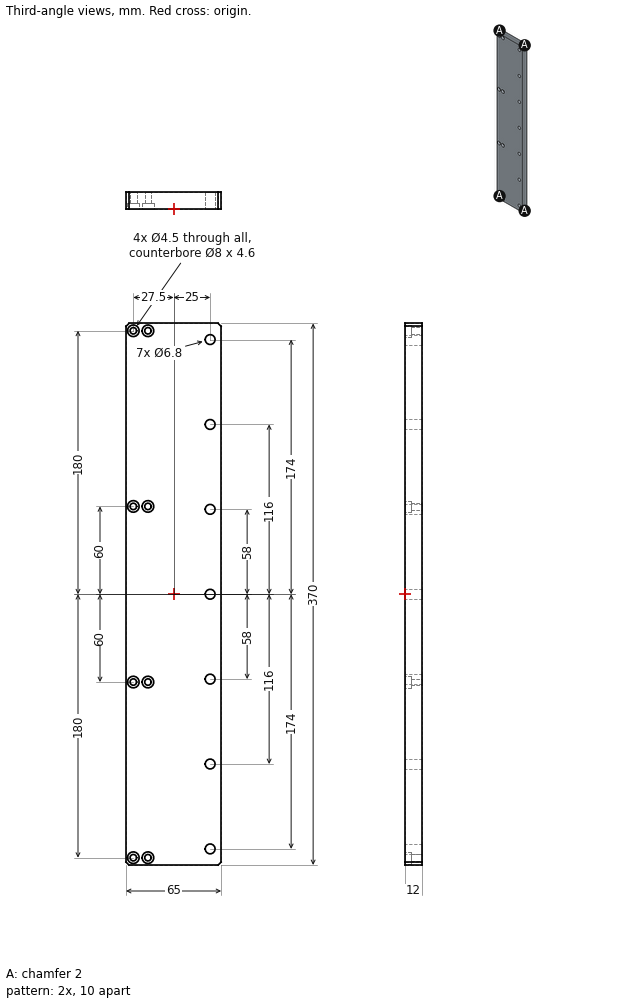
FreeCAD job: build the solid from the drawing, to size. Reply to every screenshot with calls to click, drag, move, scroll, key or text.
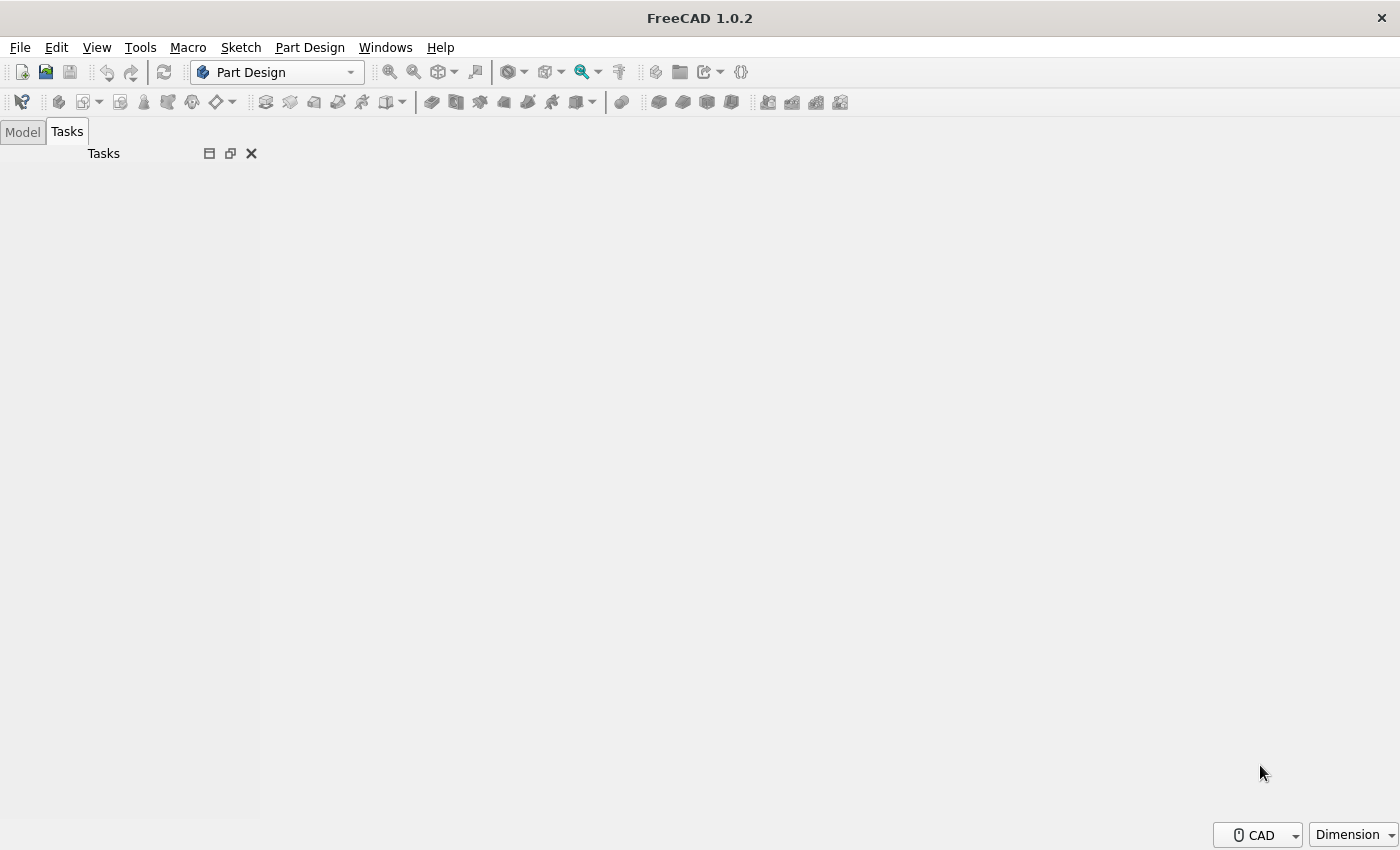
key(ctrl+n)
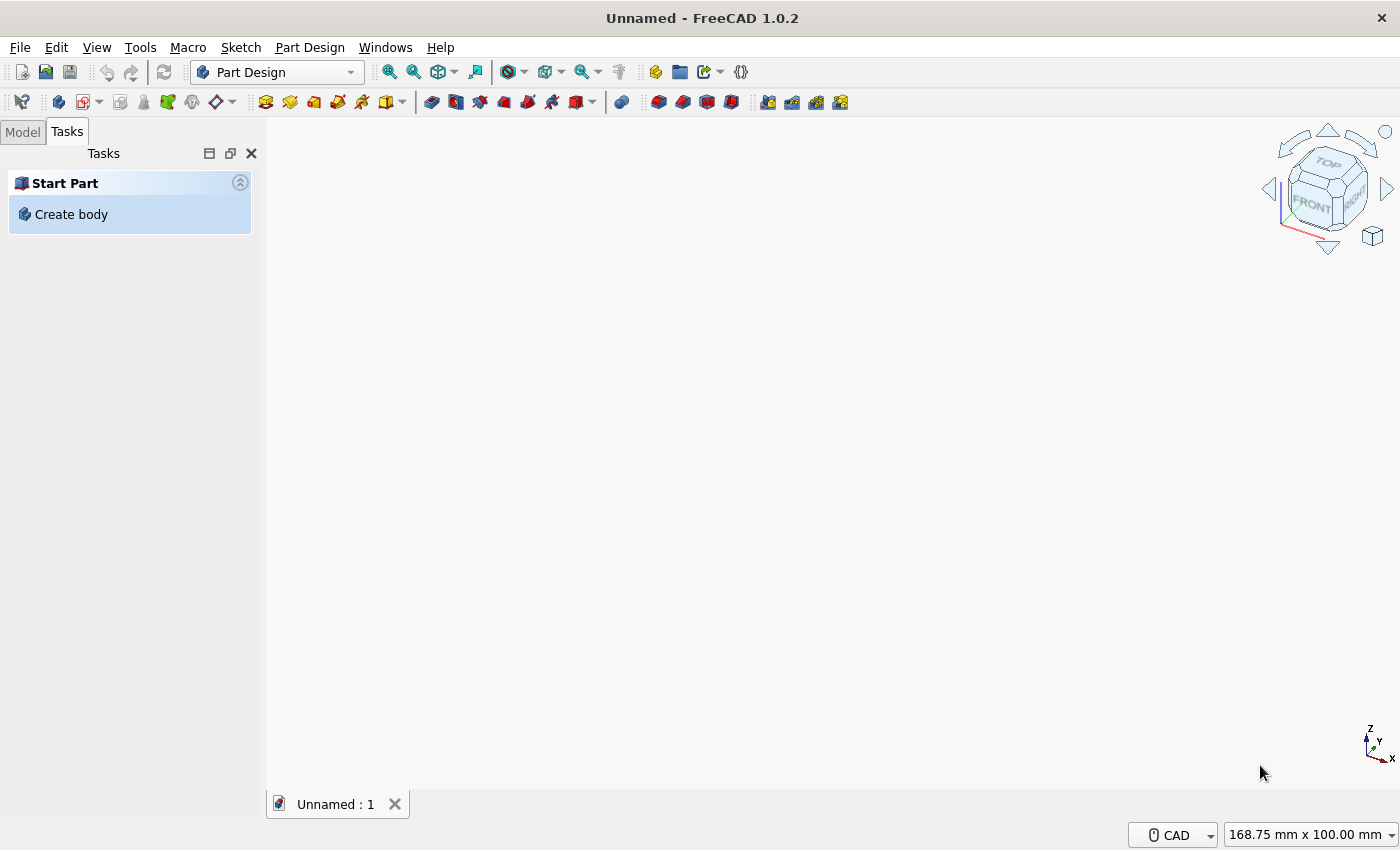
click(84, 102)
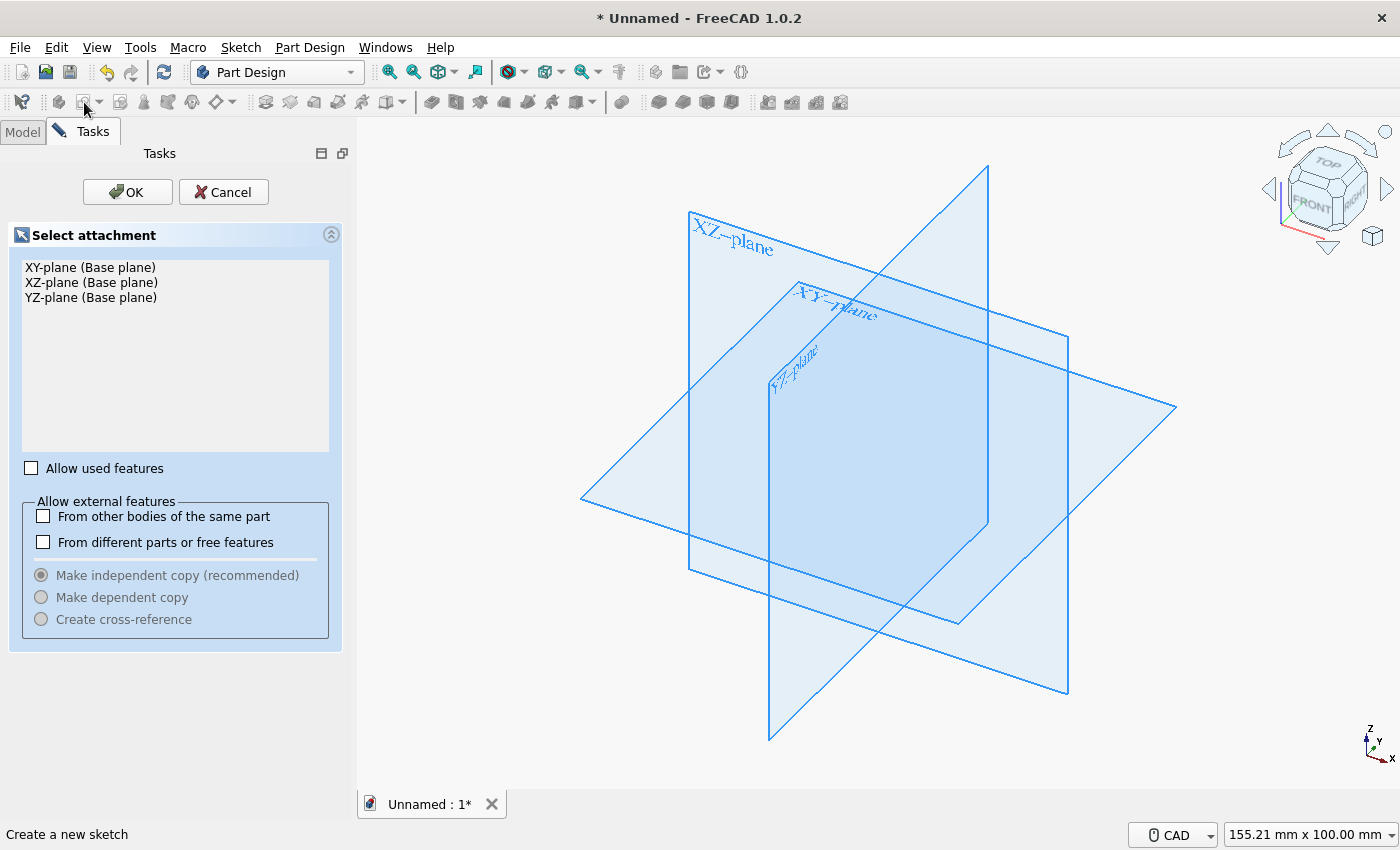
click(82, 282)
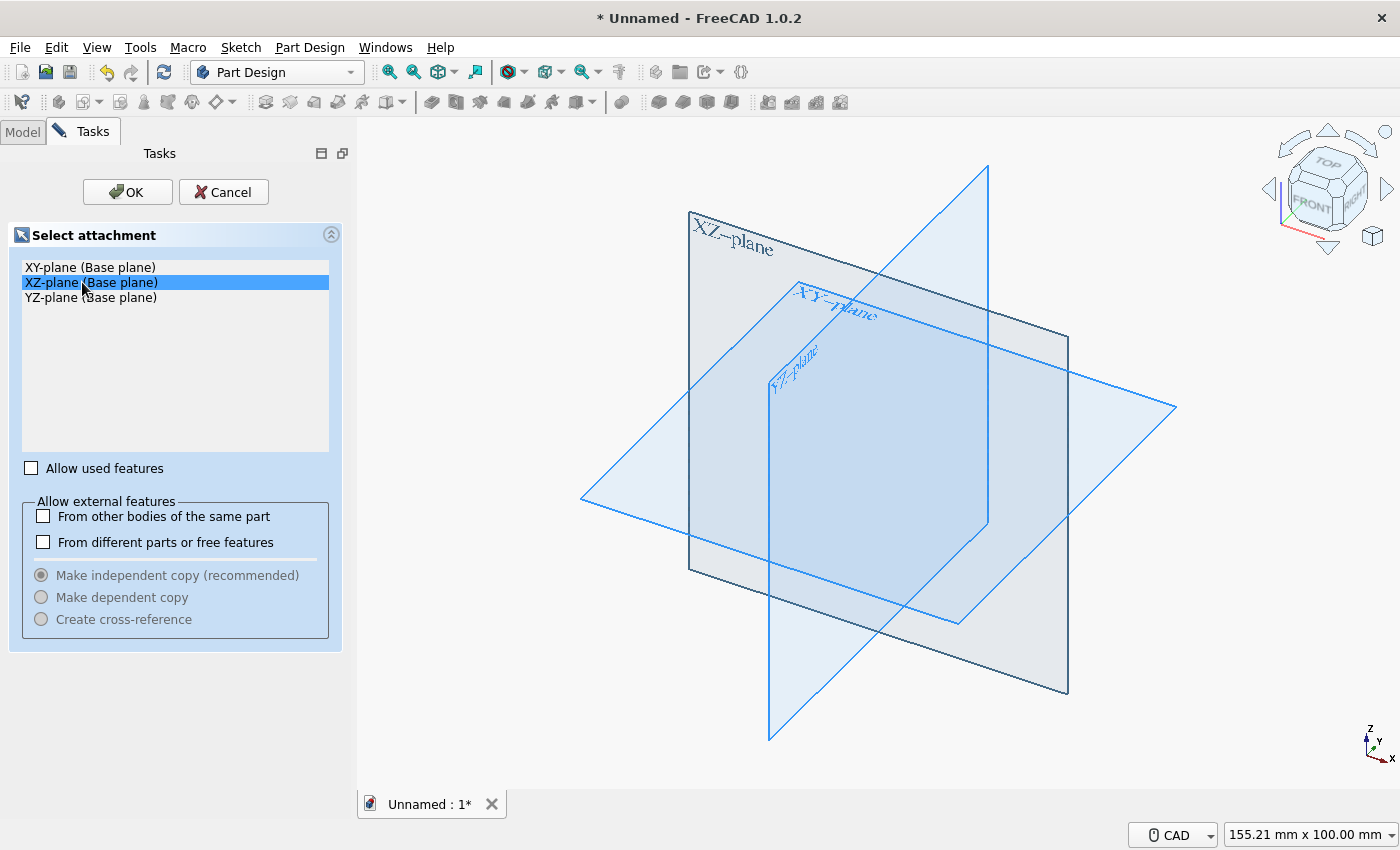
click(128, 192)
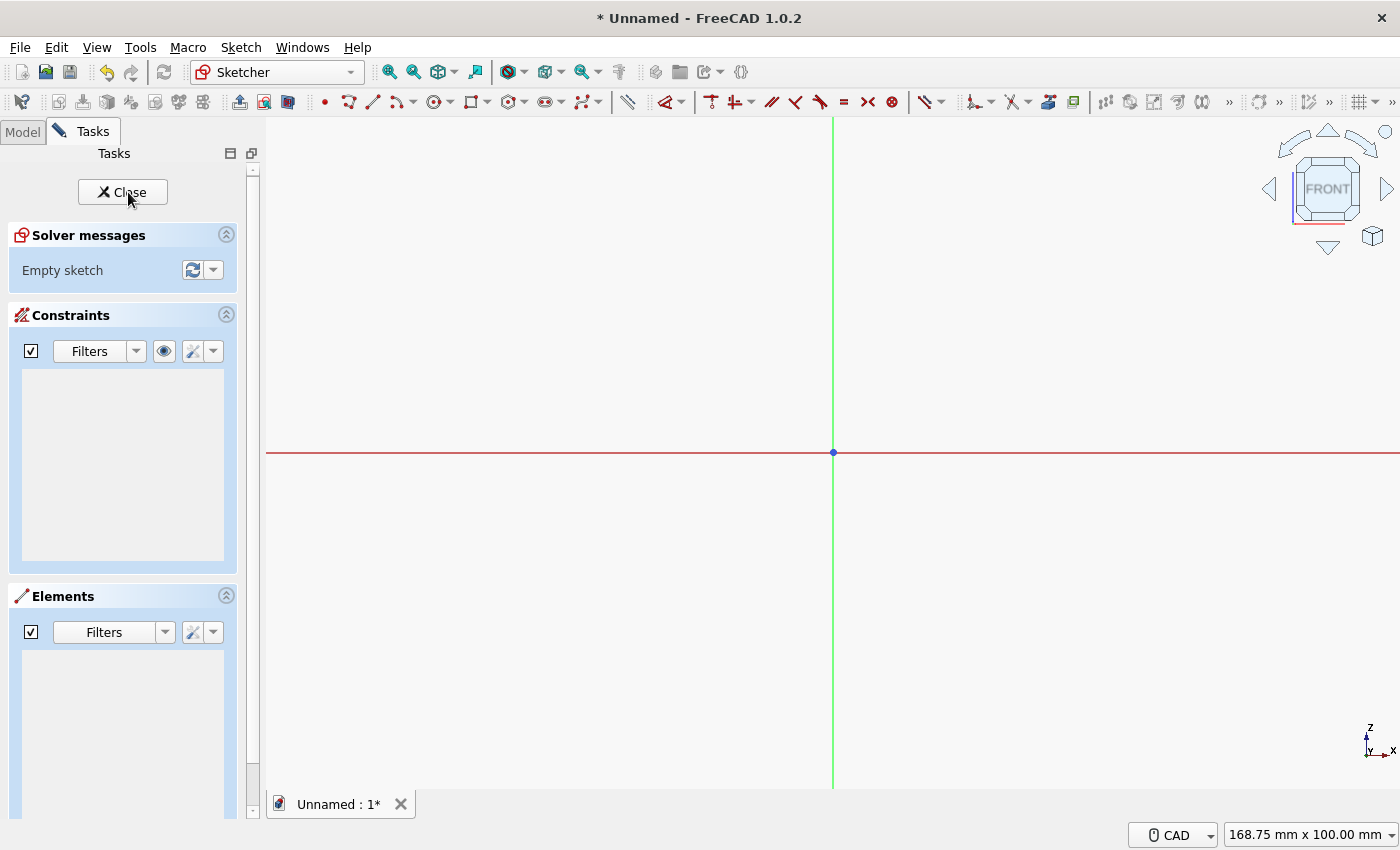
scroll(751, 453, down, 9)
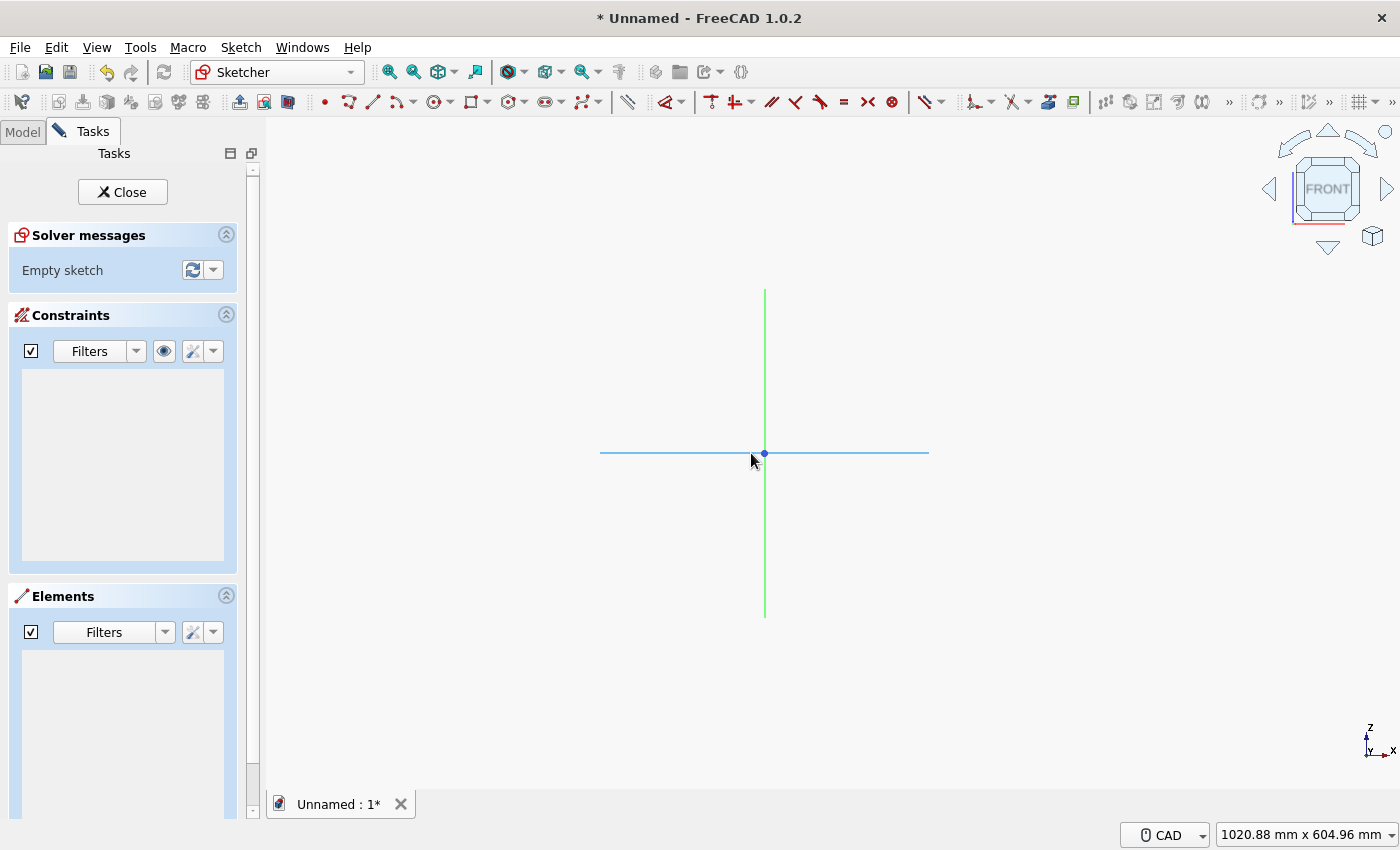
key(g)
key(v)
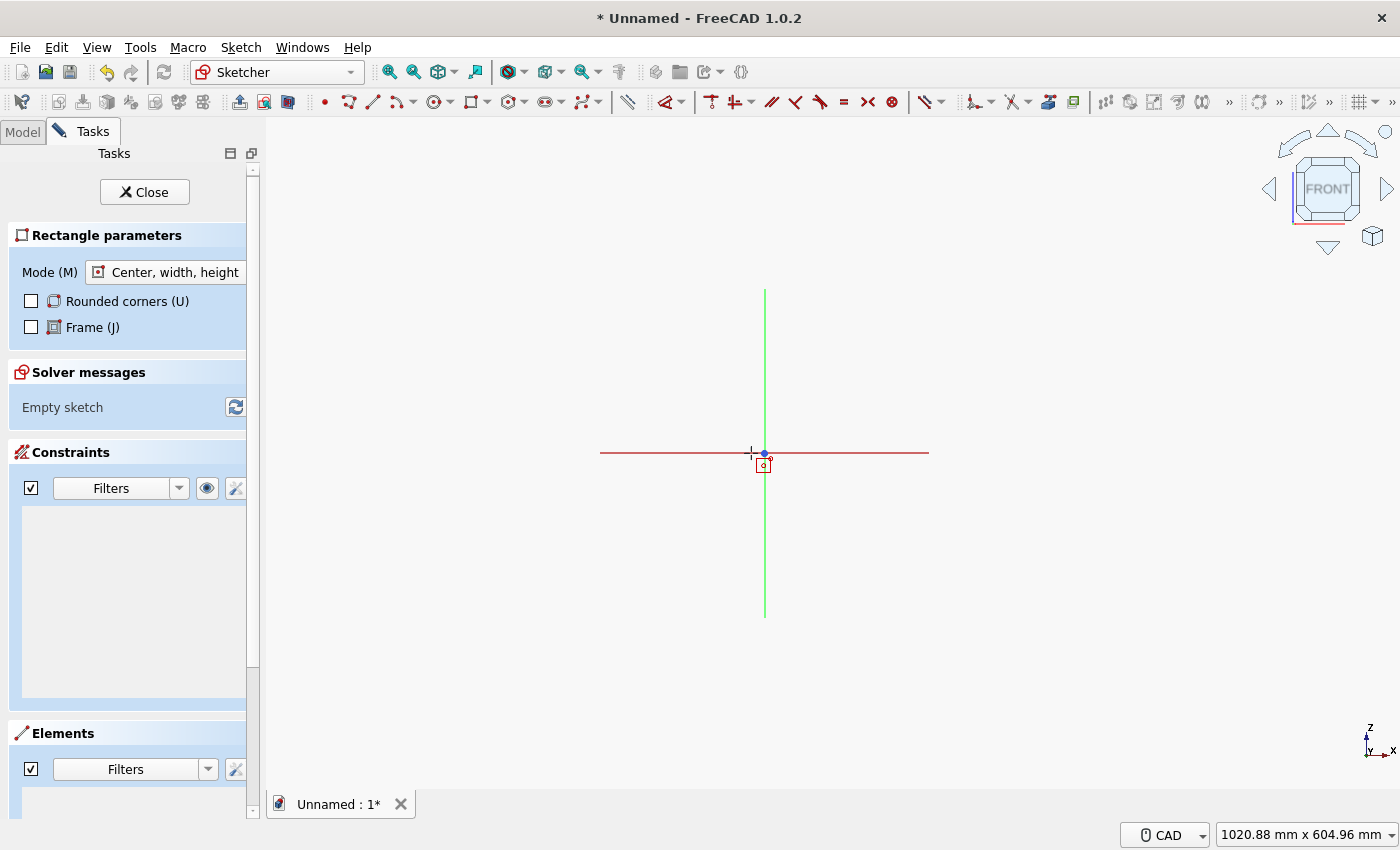
click(765, 453)
move(801, 248)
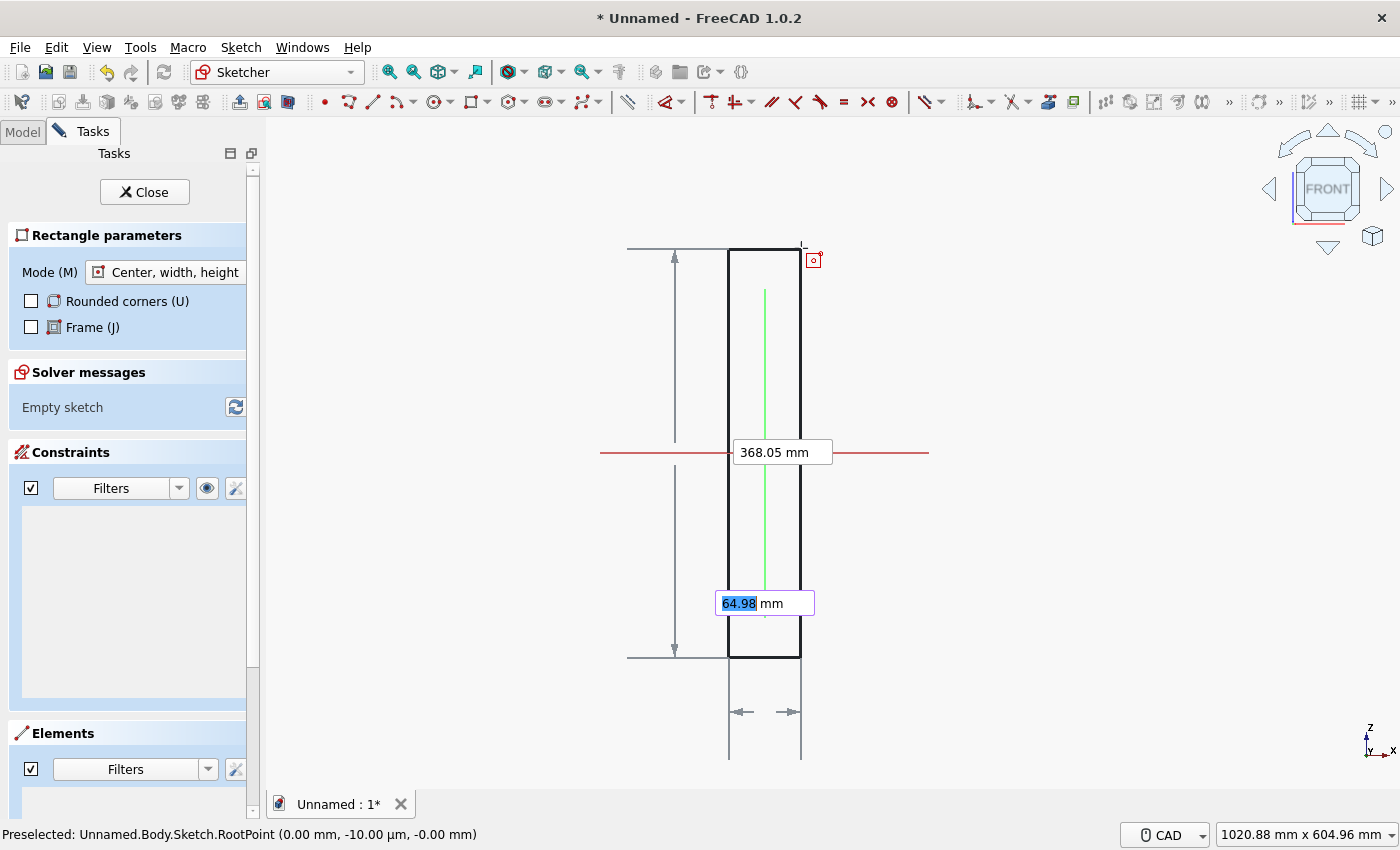
text(65)
key(Tab)
text(370)
key(Return)
key(Escape)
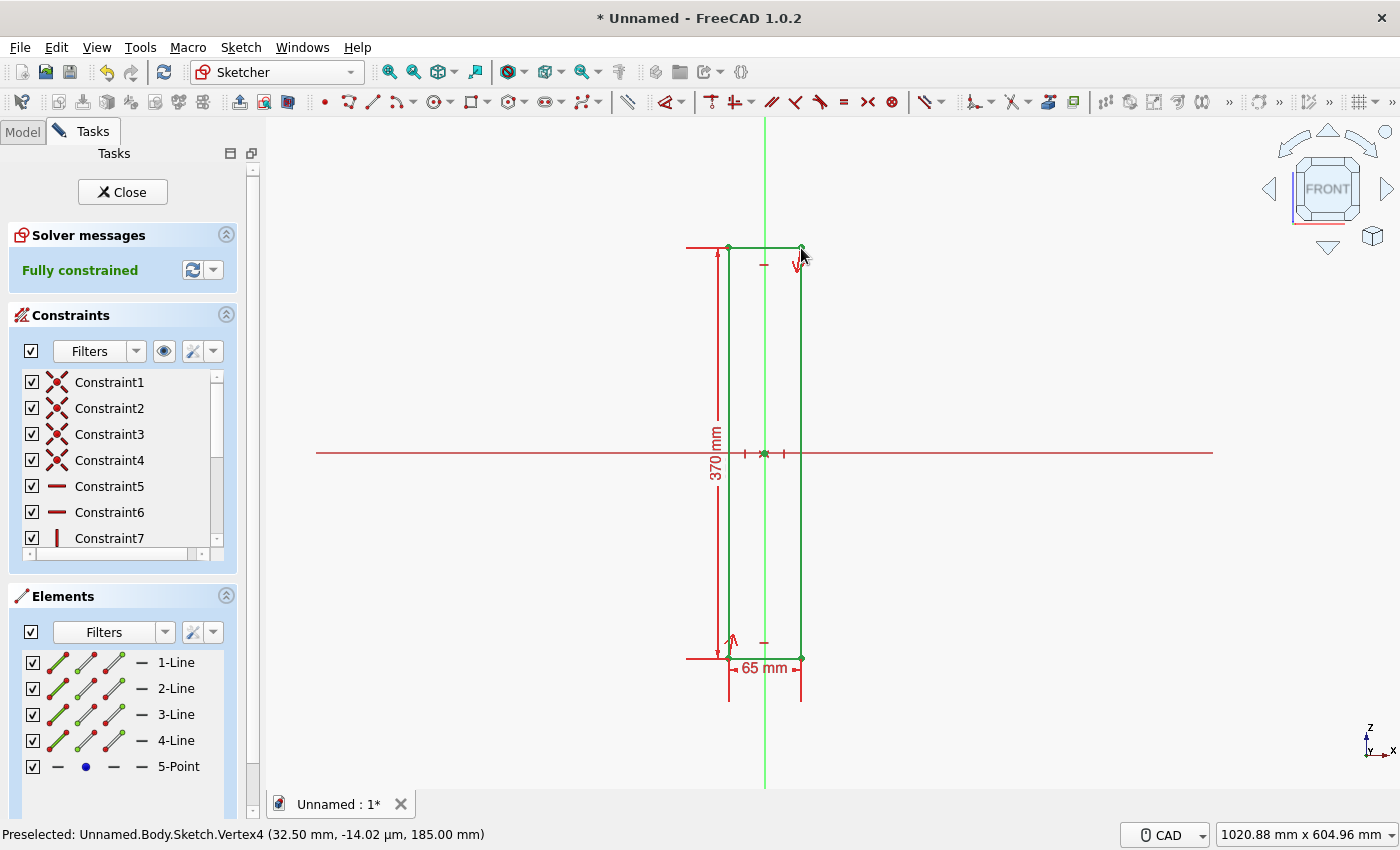
click(123, 192)